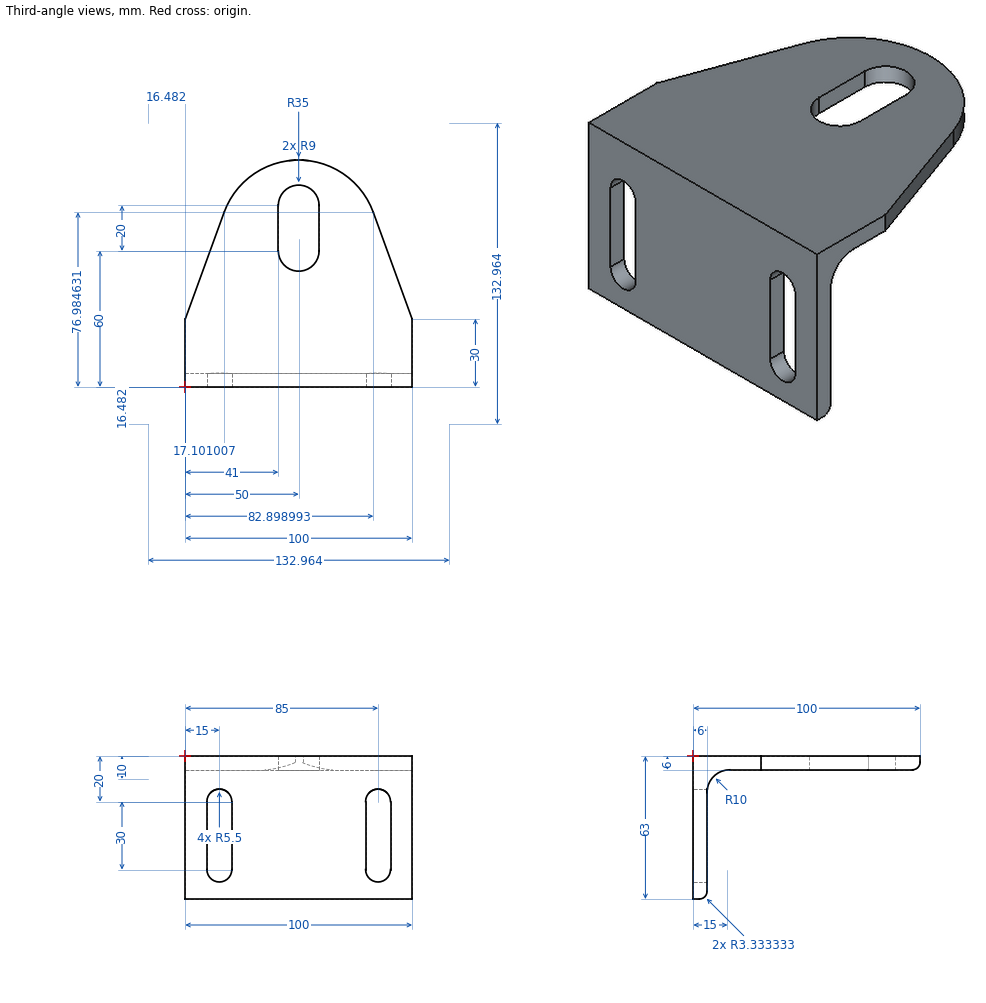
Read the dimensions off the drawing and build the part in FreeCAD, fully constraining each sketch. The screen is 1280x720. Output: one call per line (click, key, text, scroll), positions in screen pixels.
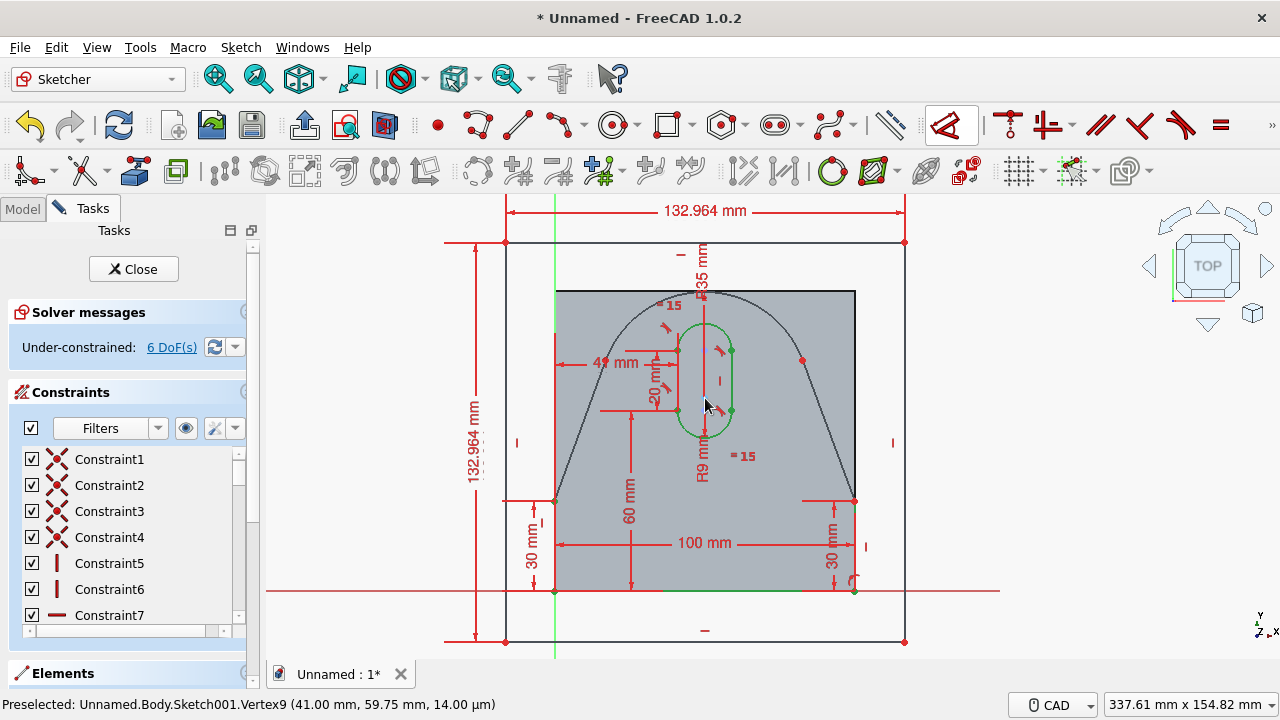
click(704, 397)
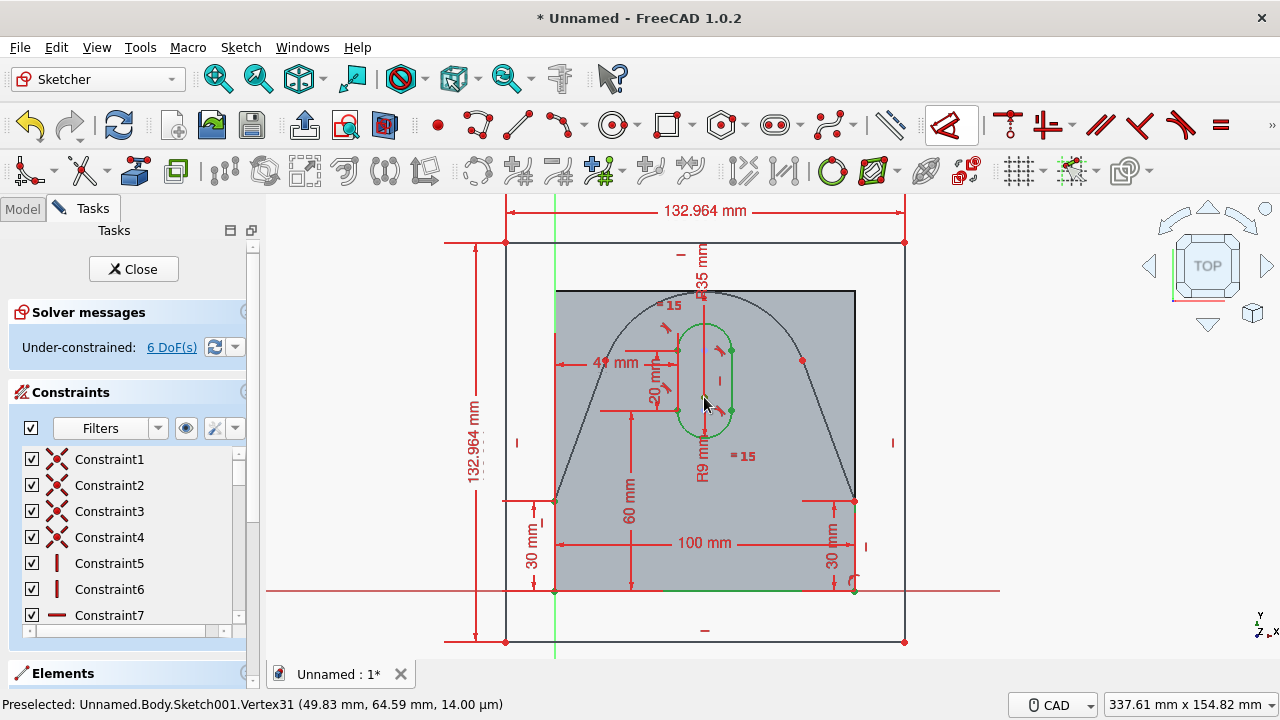
click(972, 126)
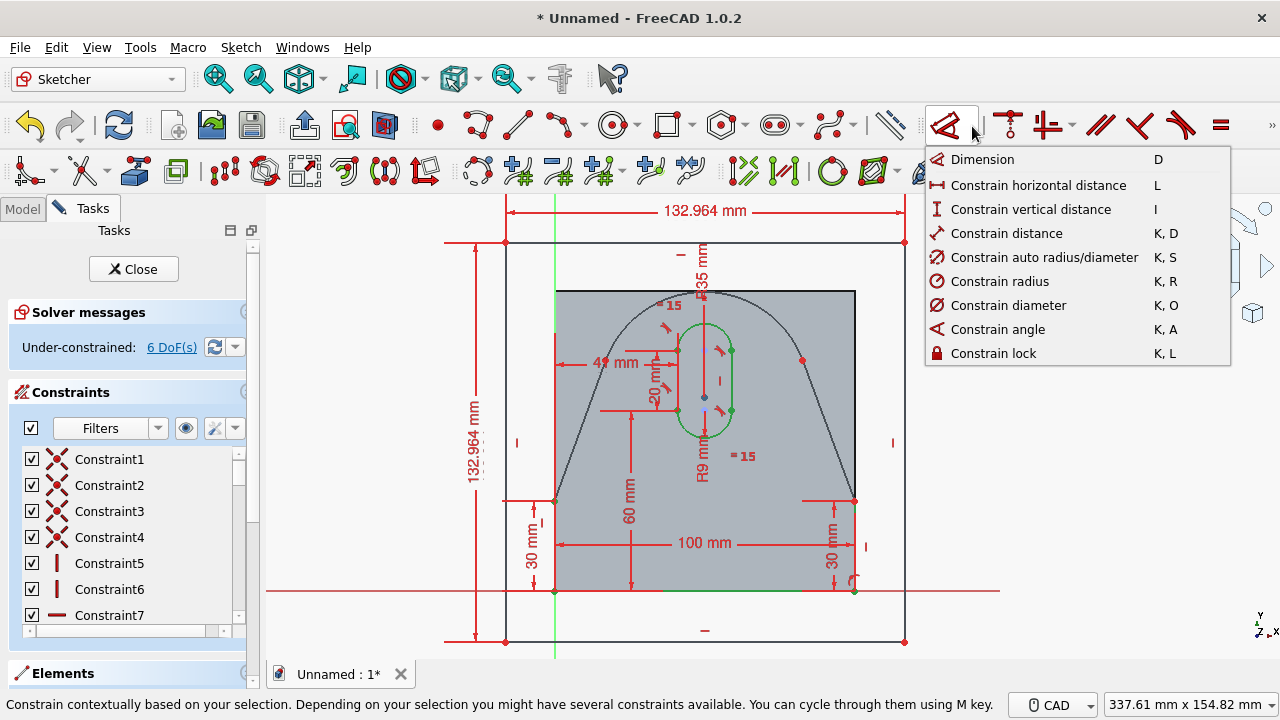
click(1078, 185)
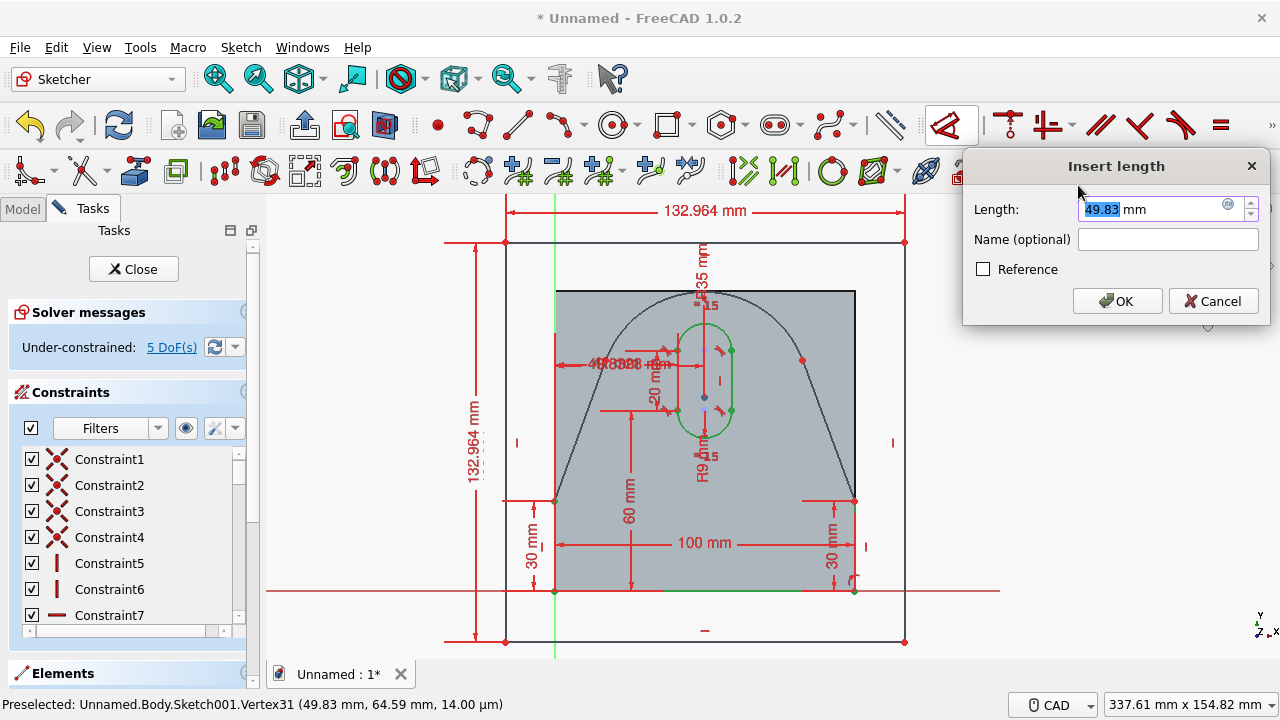
text(50)
key(Return)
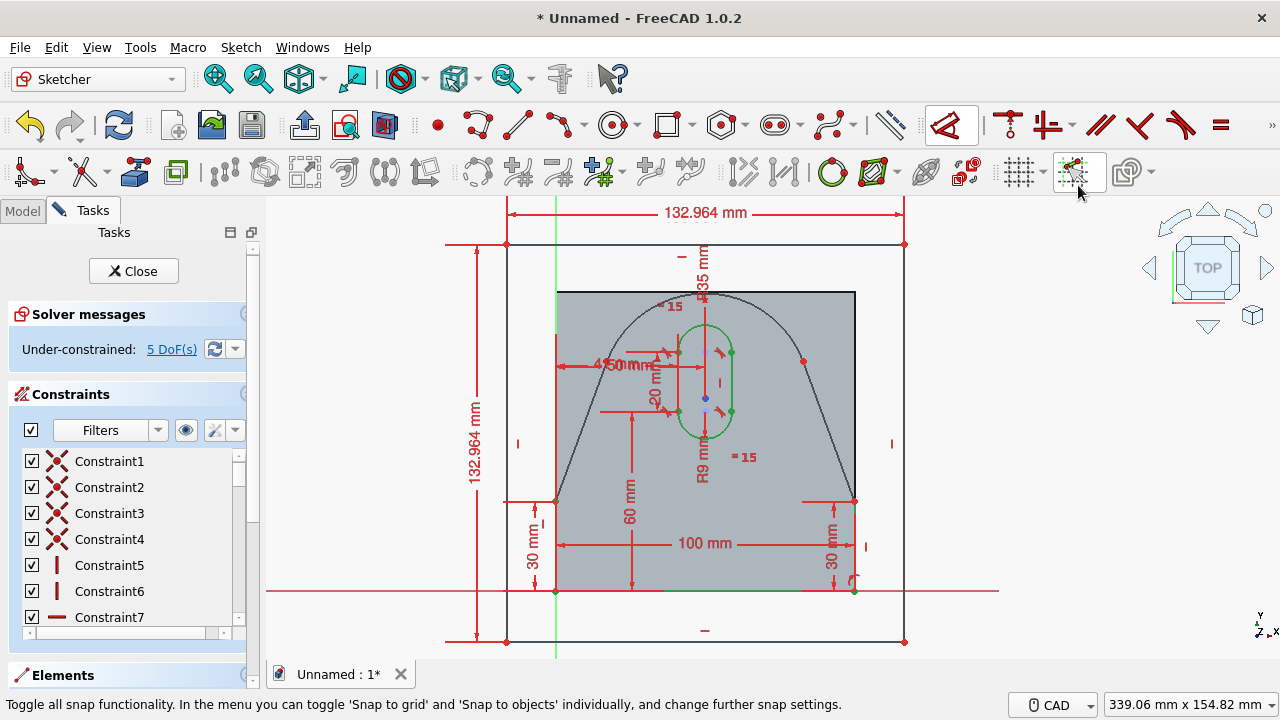
click(507, 245)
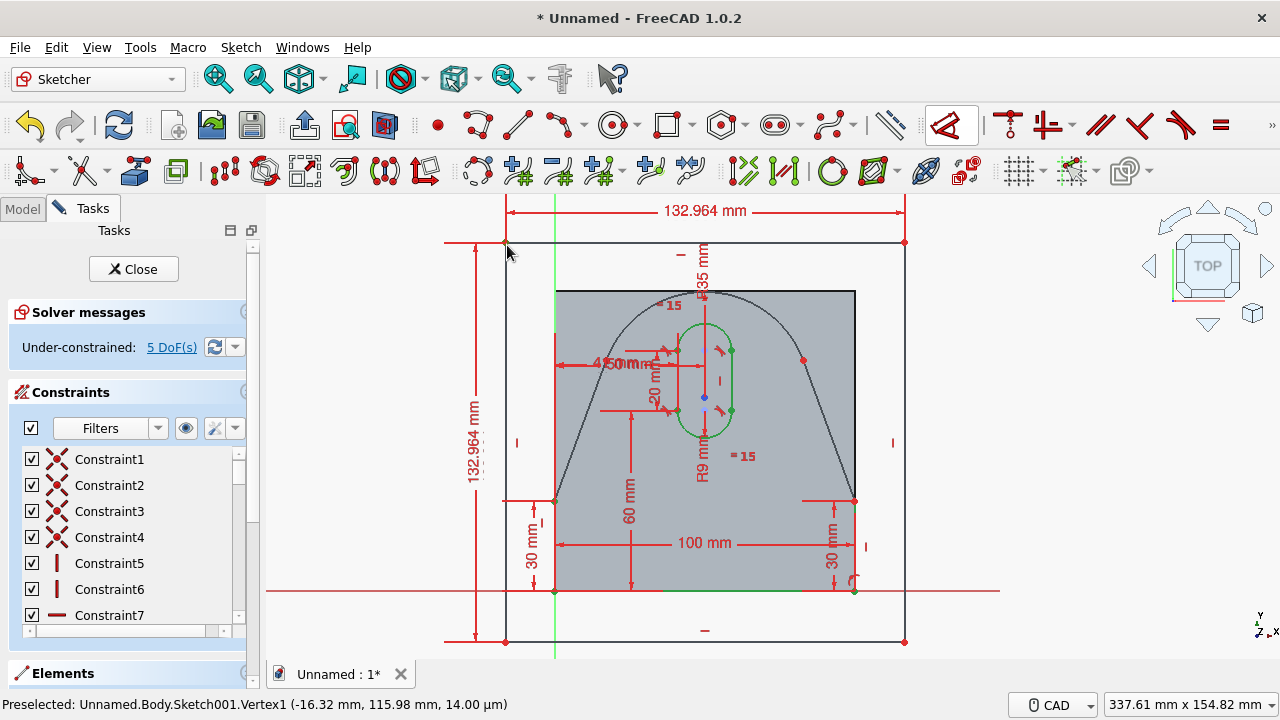
key(l)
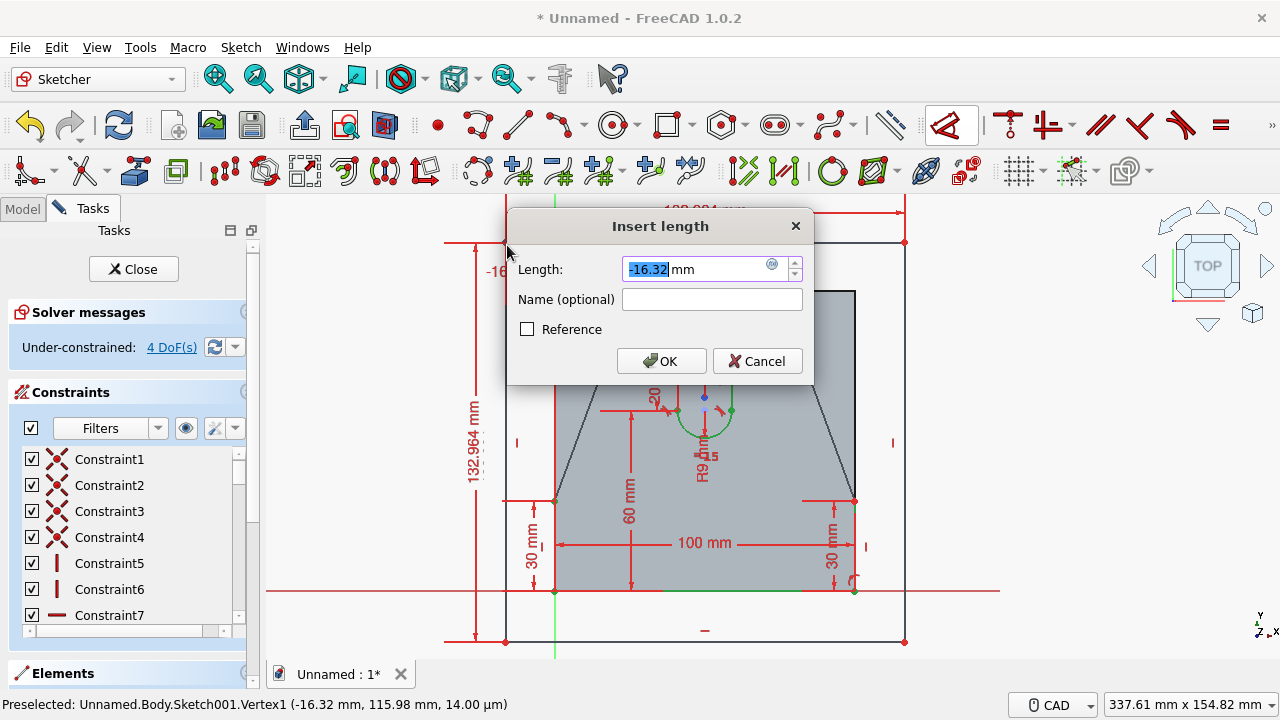
text(-16.482)
key(Return)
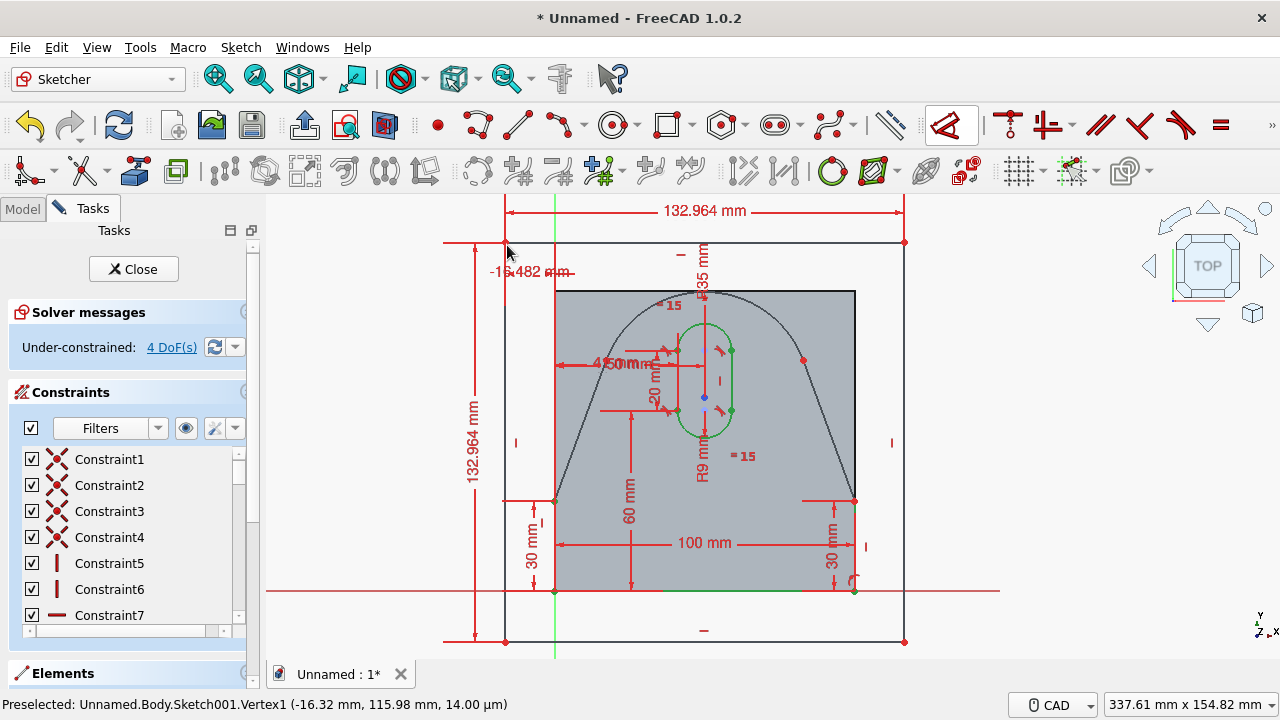
scroll(704, 397, down, 2)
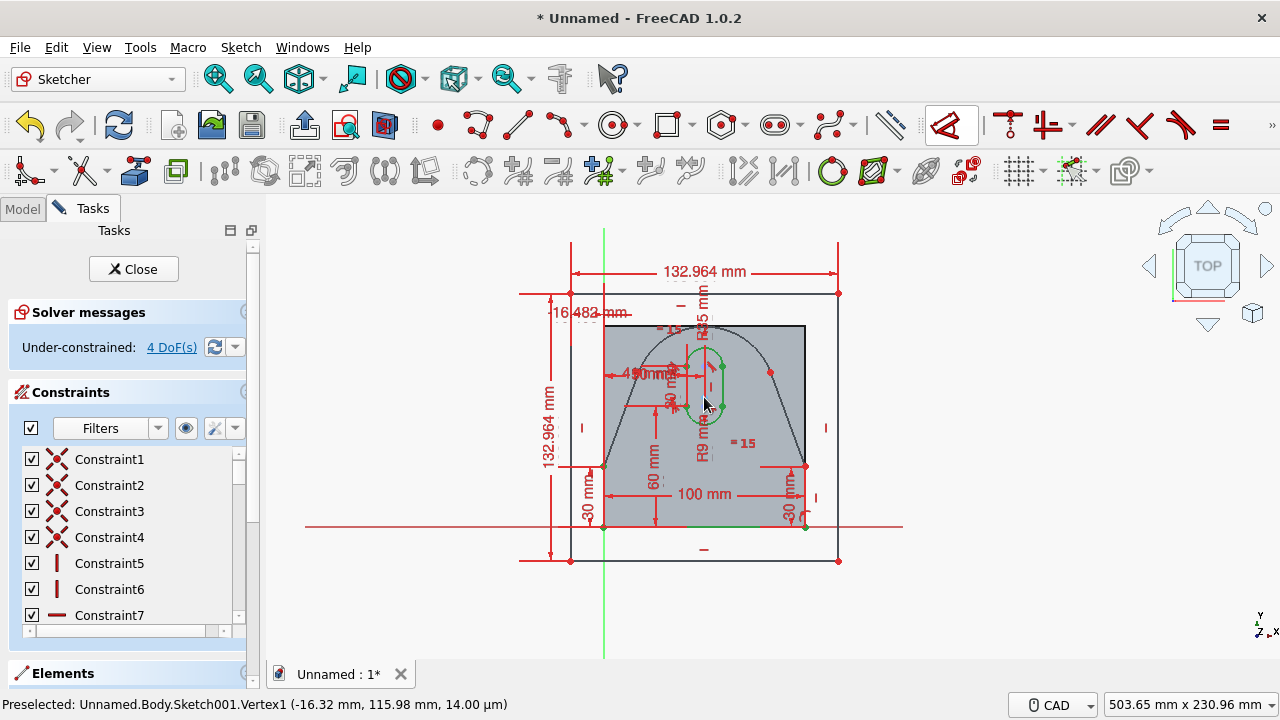
click(571, 561)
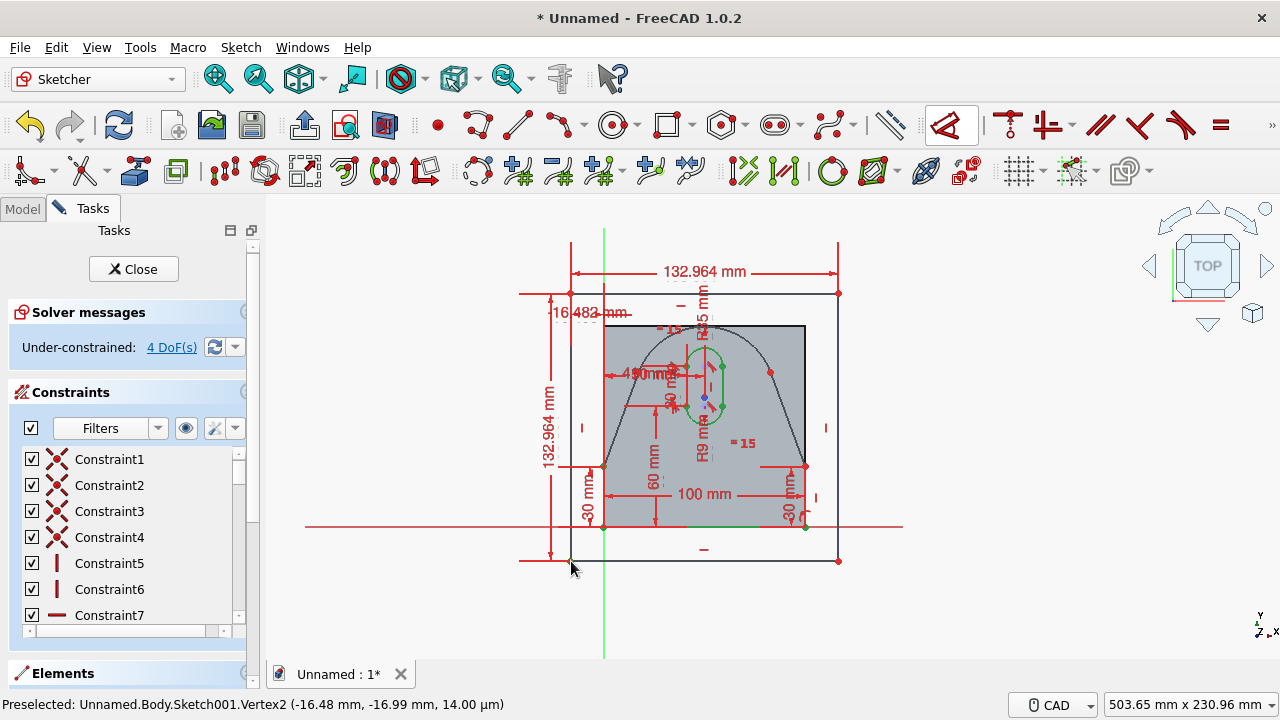
key(i)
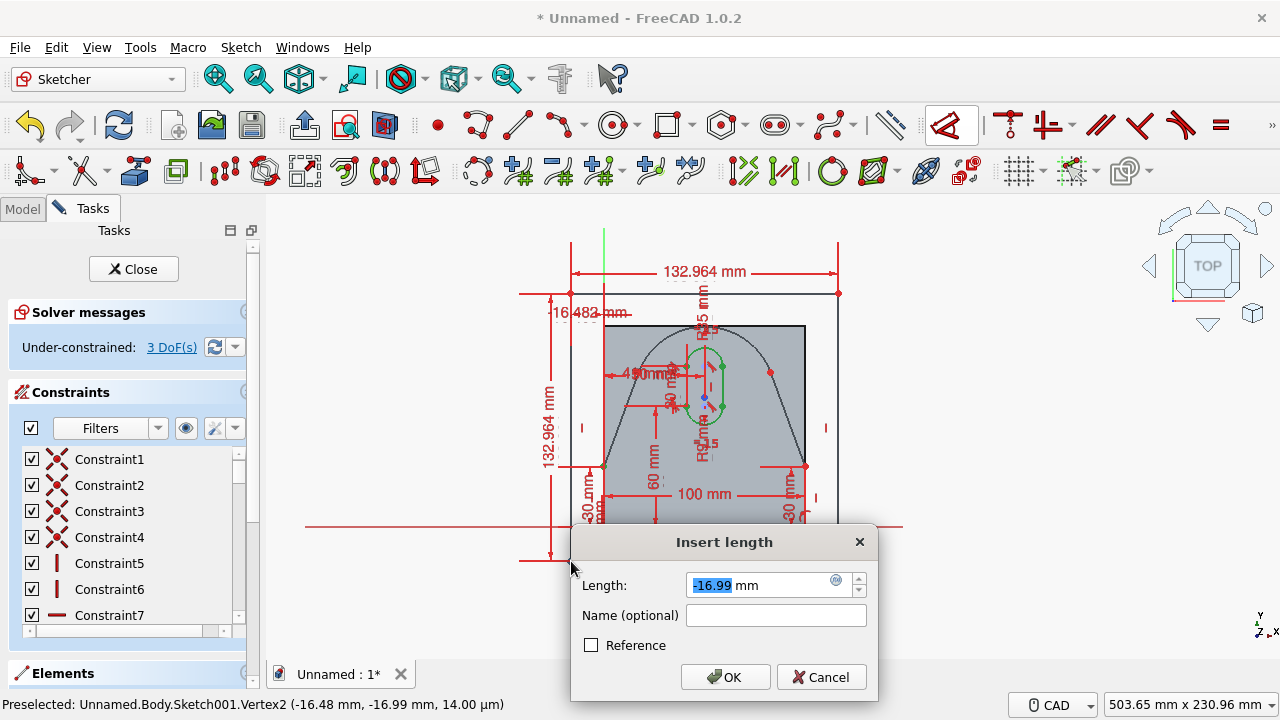
text(-16.482)
key(Return)